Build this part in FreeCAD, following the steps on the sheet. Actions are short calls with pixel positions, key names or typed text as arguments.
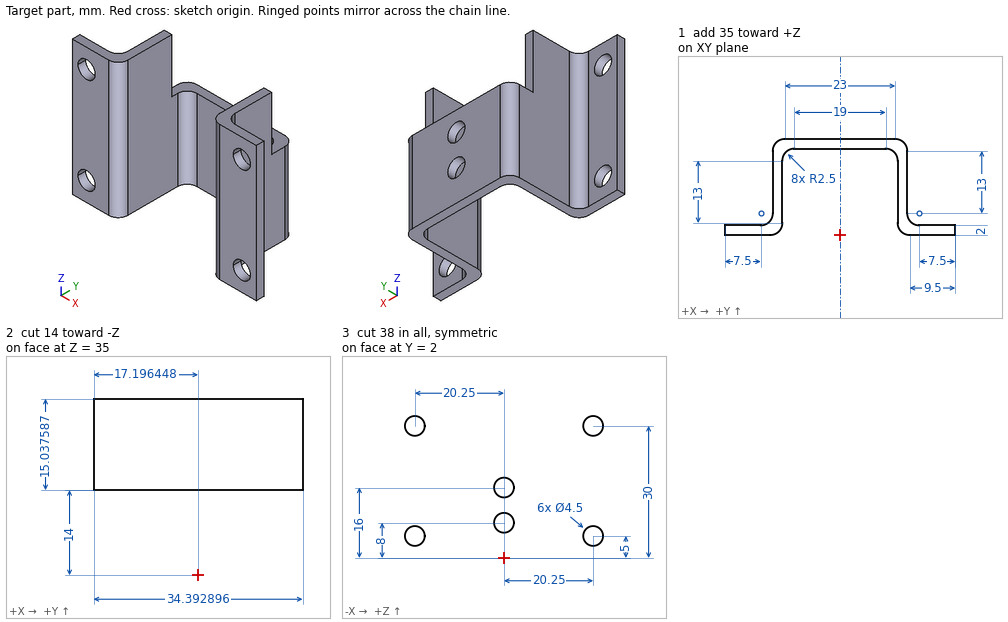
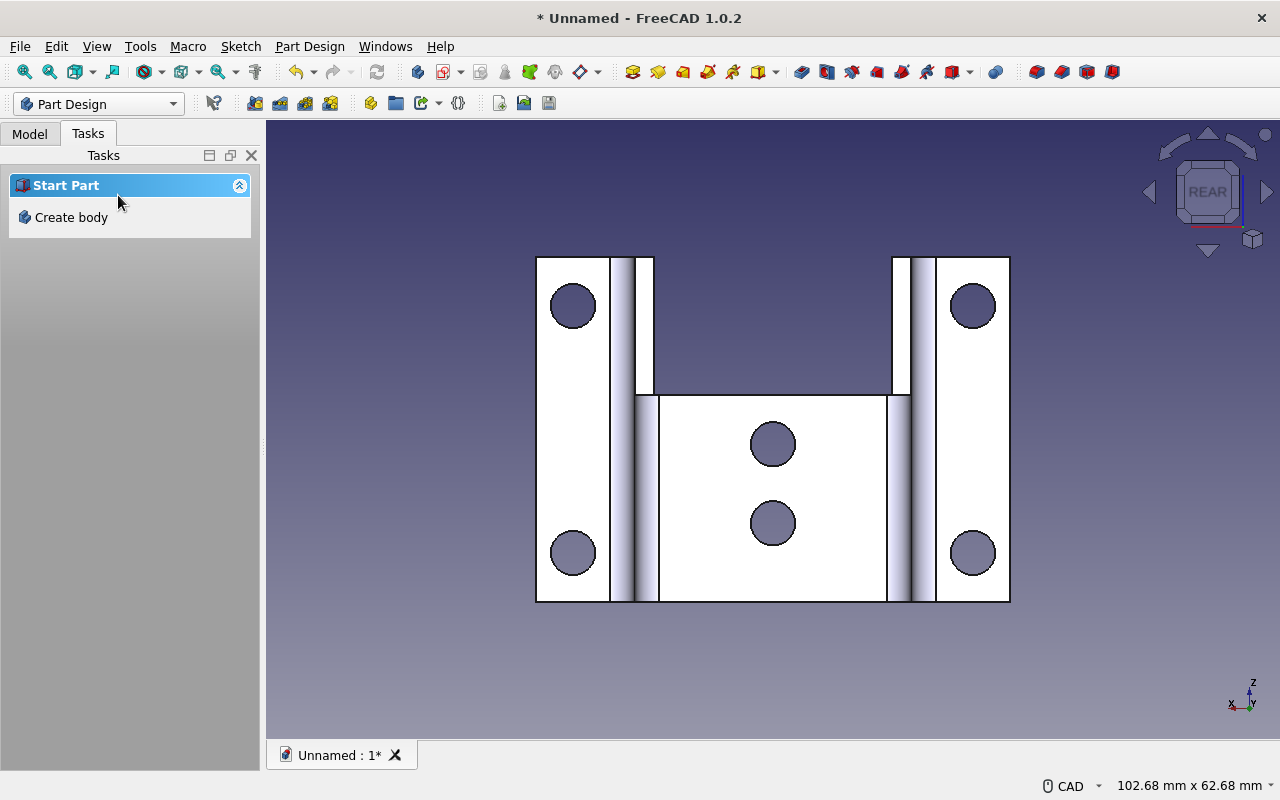
key(0)